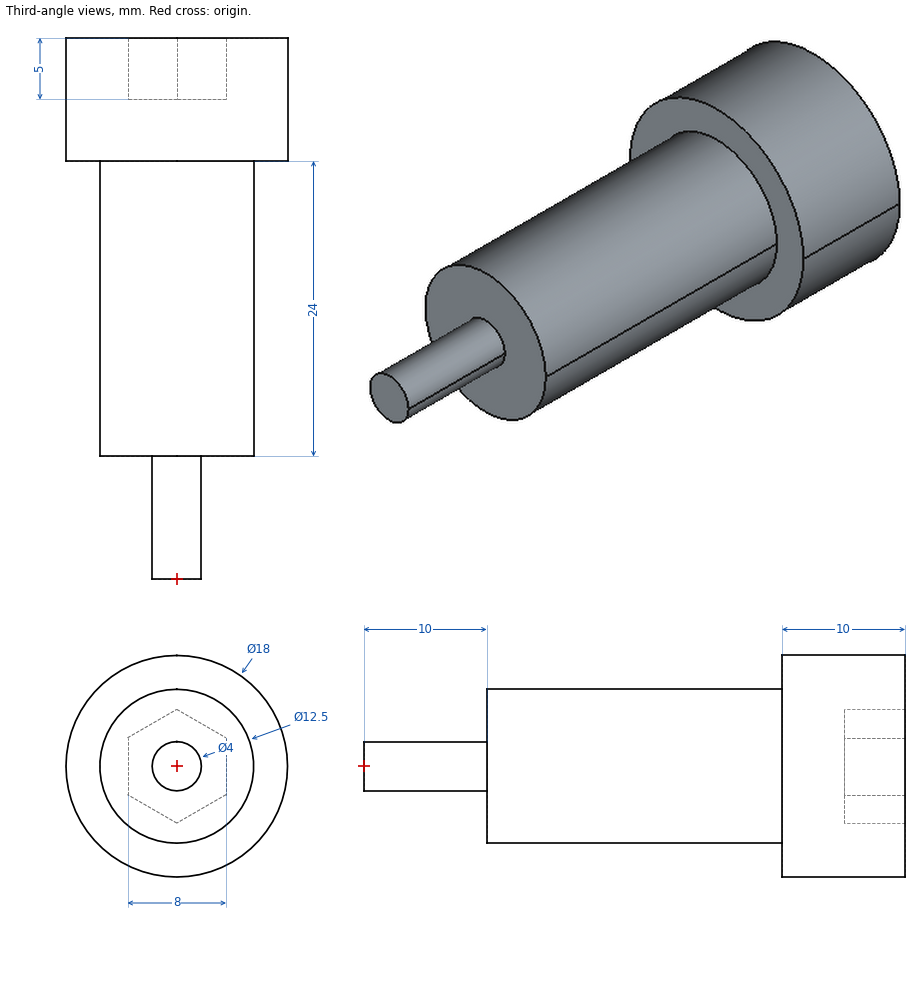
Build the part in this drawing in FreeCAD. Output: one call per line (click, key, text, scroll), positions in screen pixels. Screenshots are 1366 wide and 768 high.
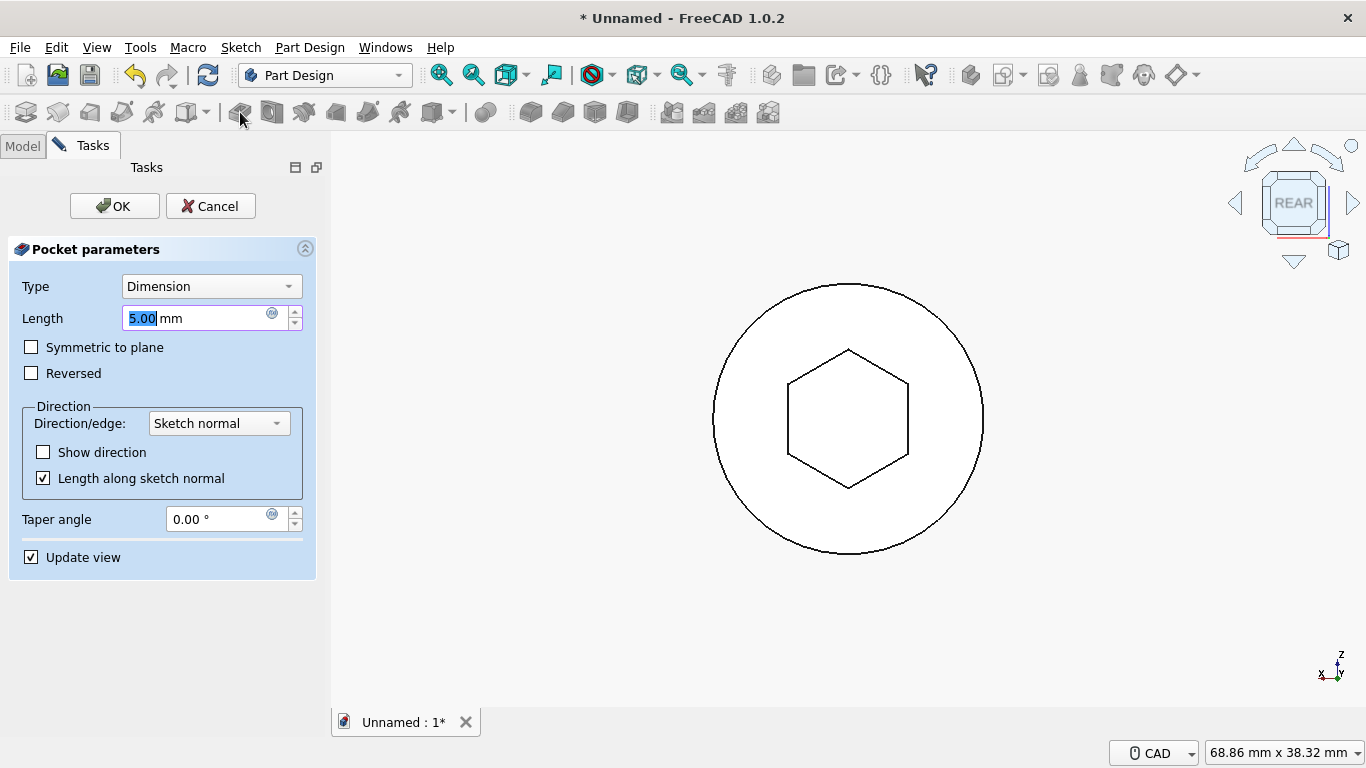
text(5)
key(Tab)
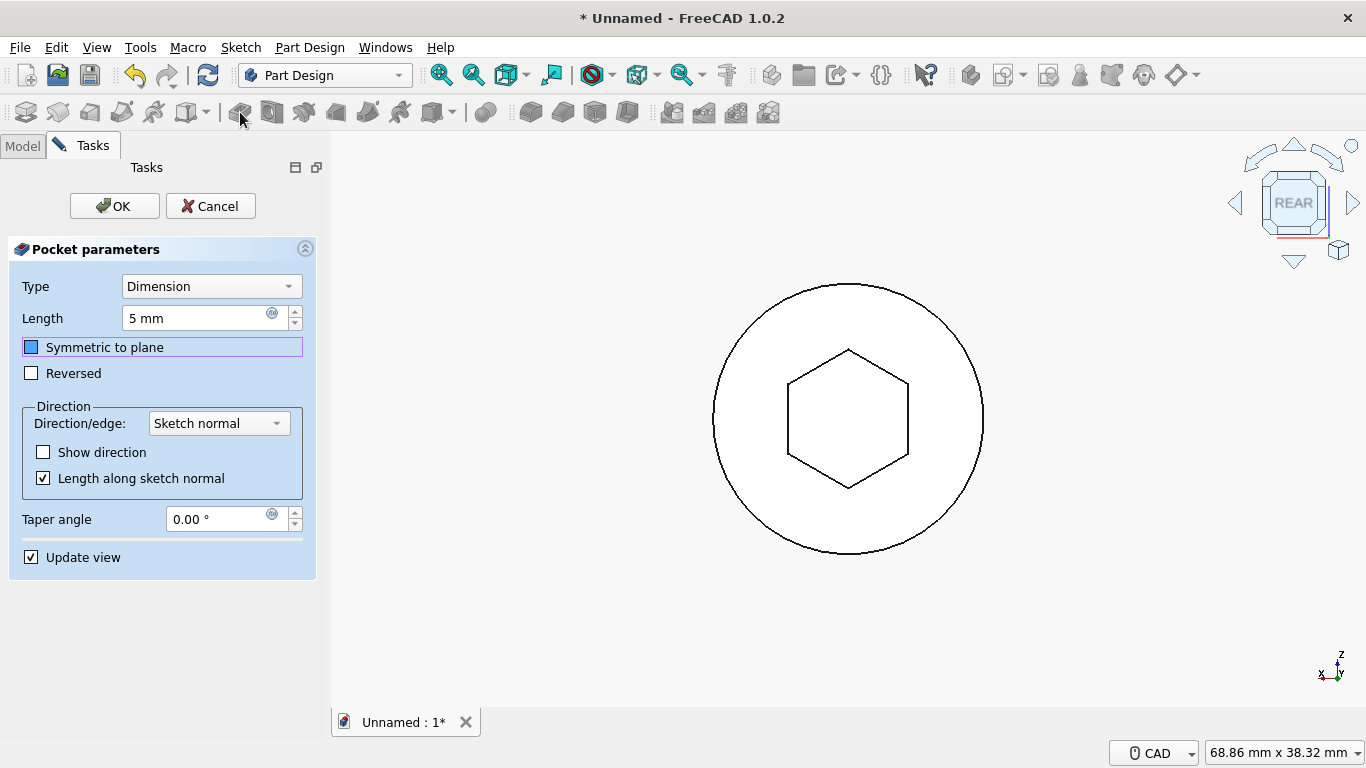
click(115, 206)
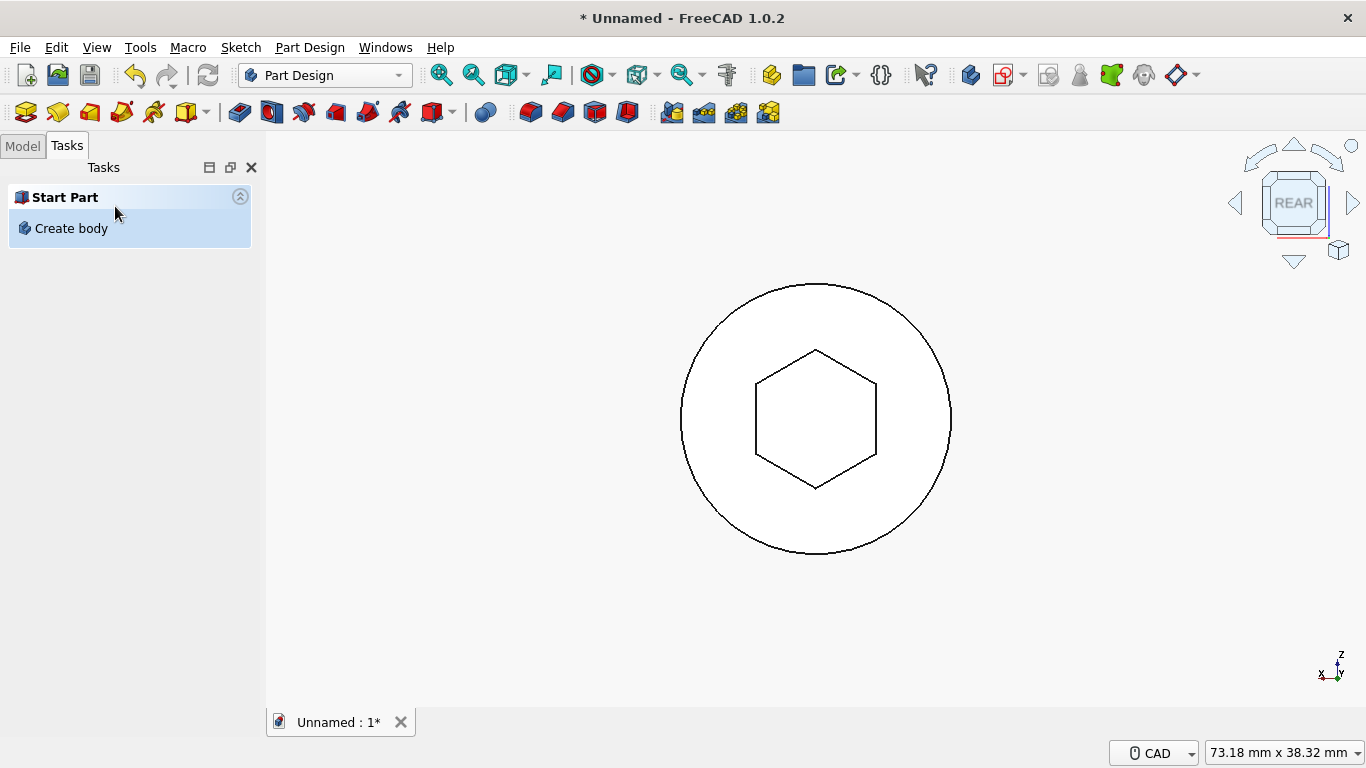
key(0)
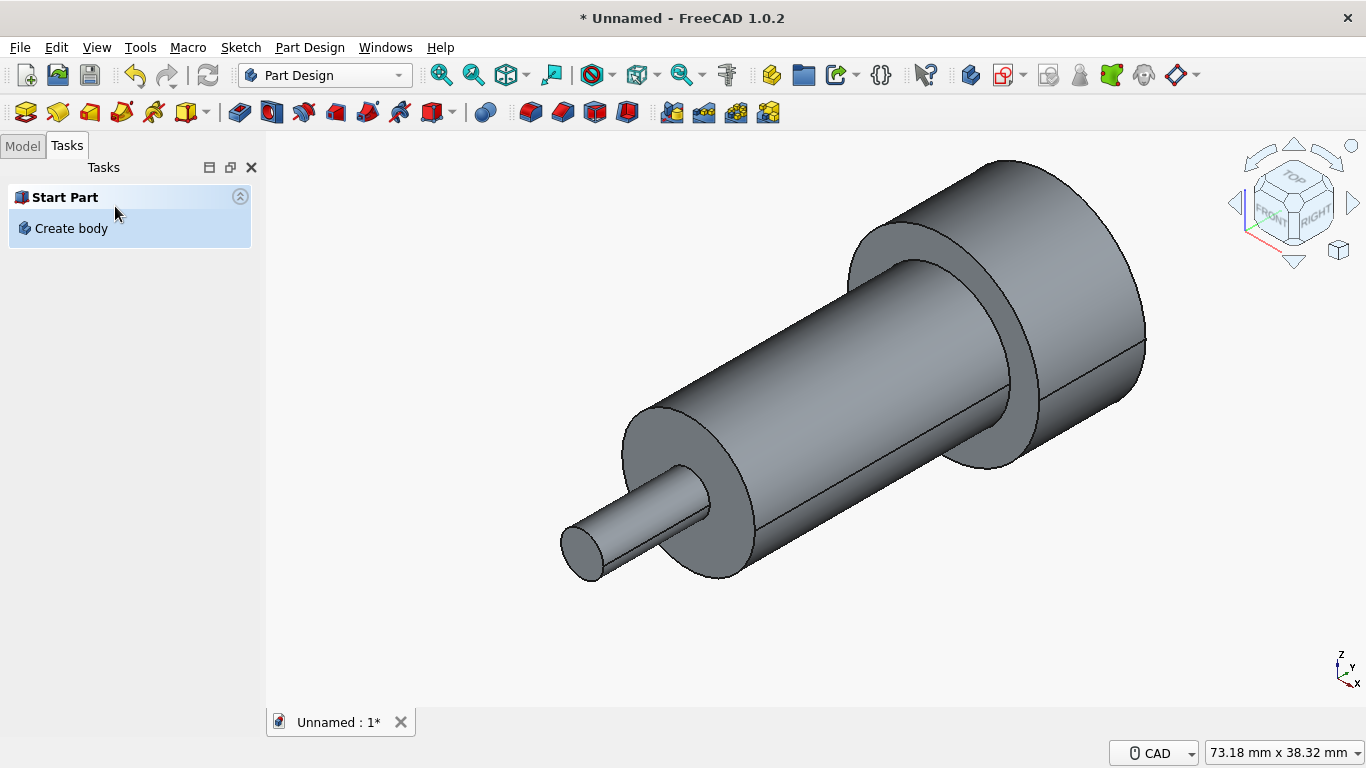
key(v)
key(f)